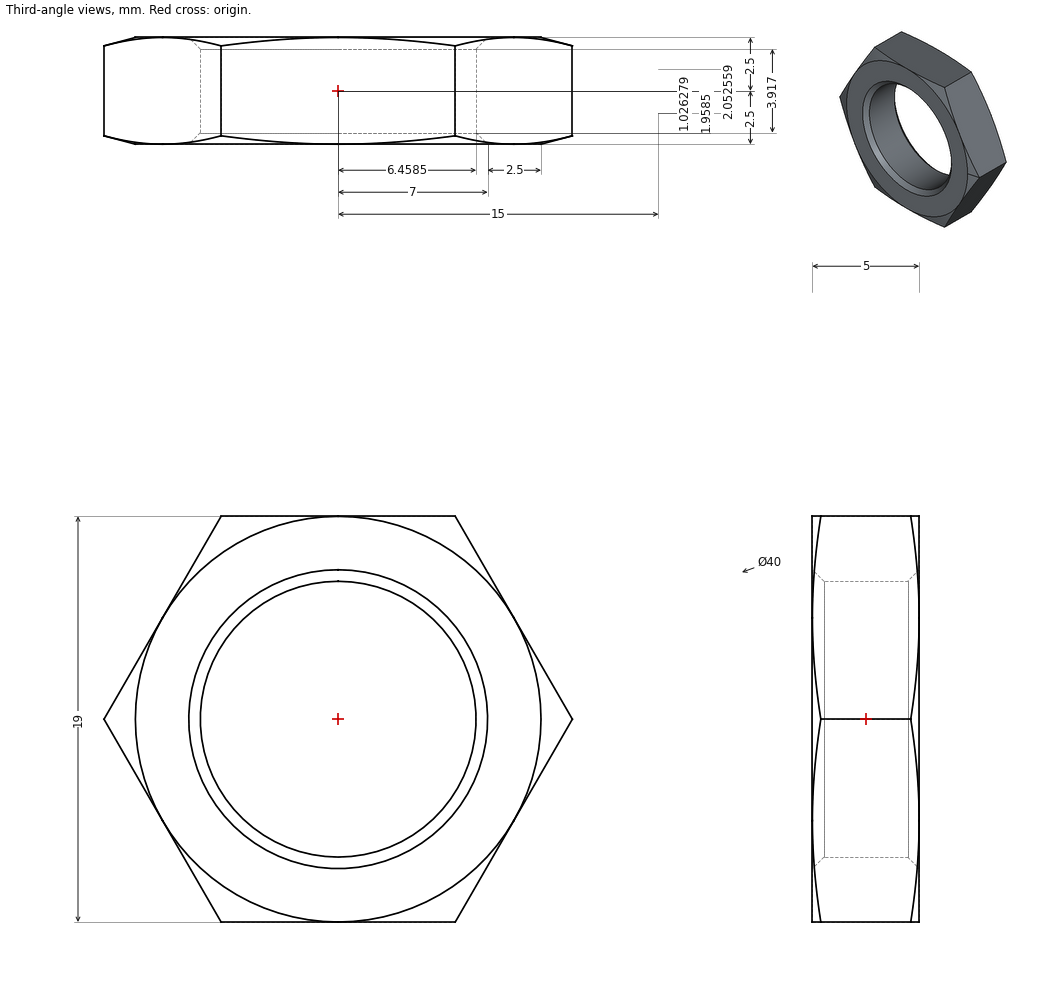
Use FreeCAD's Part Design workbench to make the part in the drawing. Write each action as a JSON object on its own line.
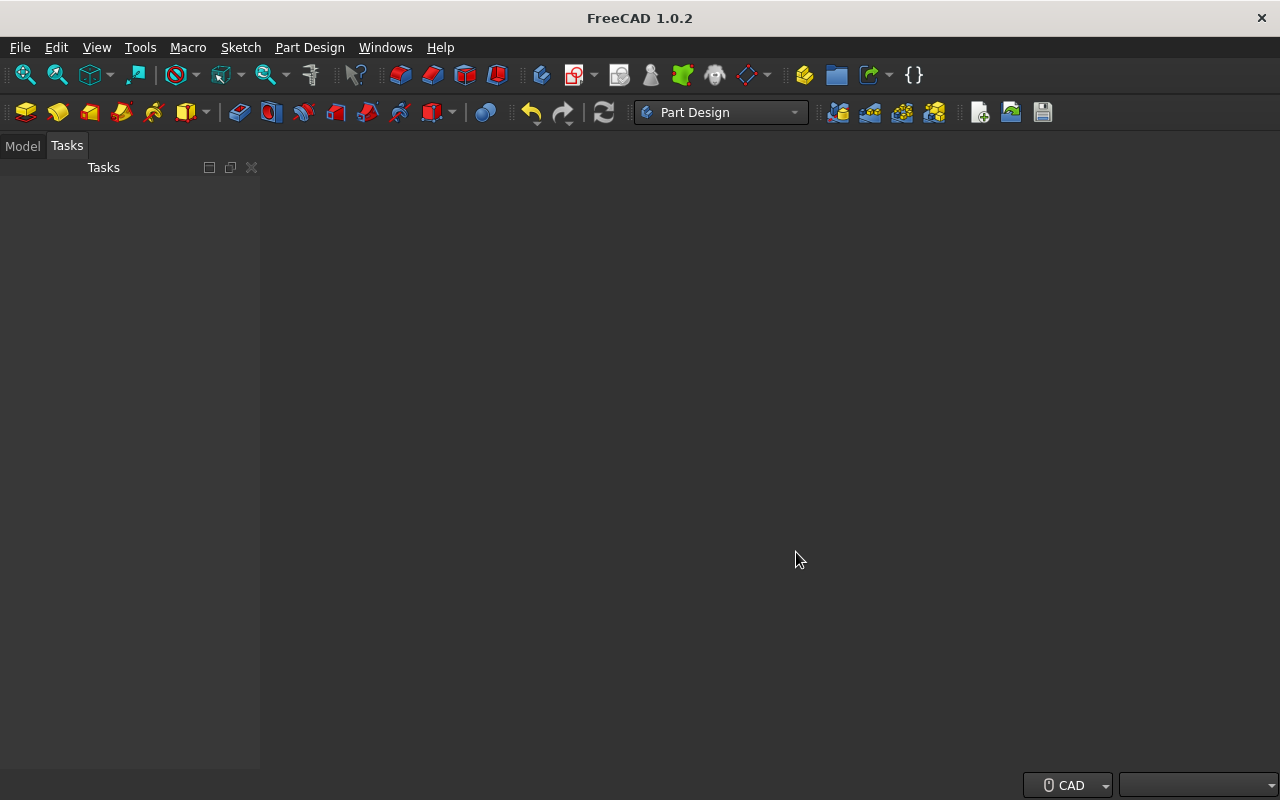
{"action": "key", "text": "ctrl+n"}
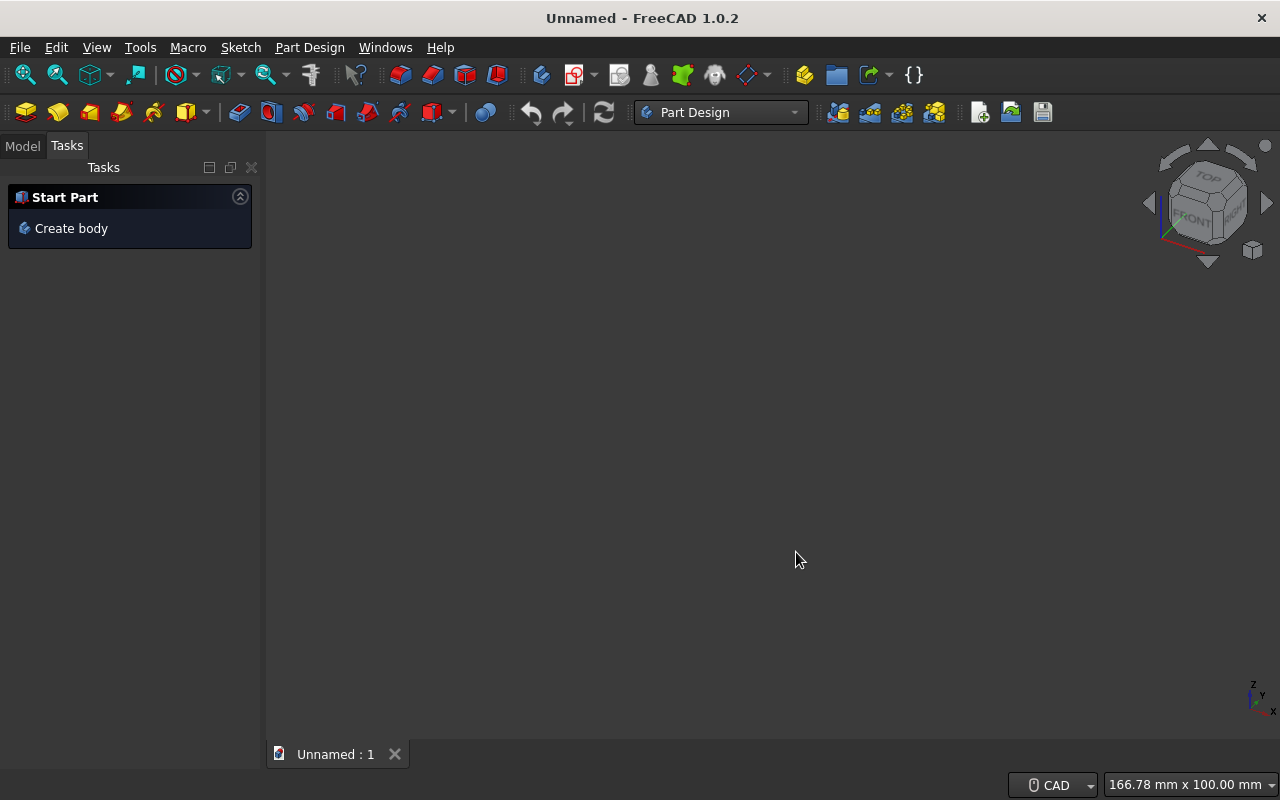
{"action": "left_click", "coordinate": [574, 76]}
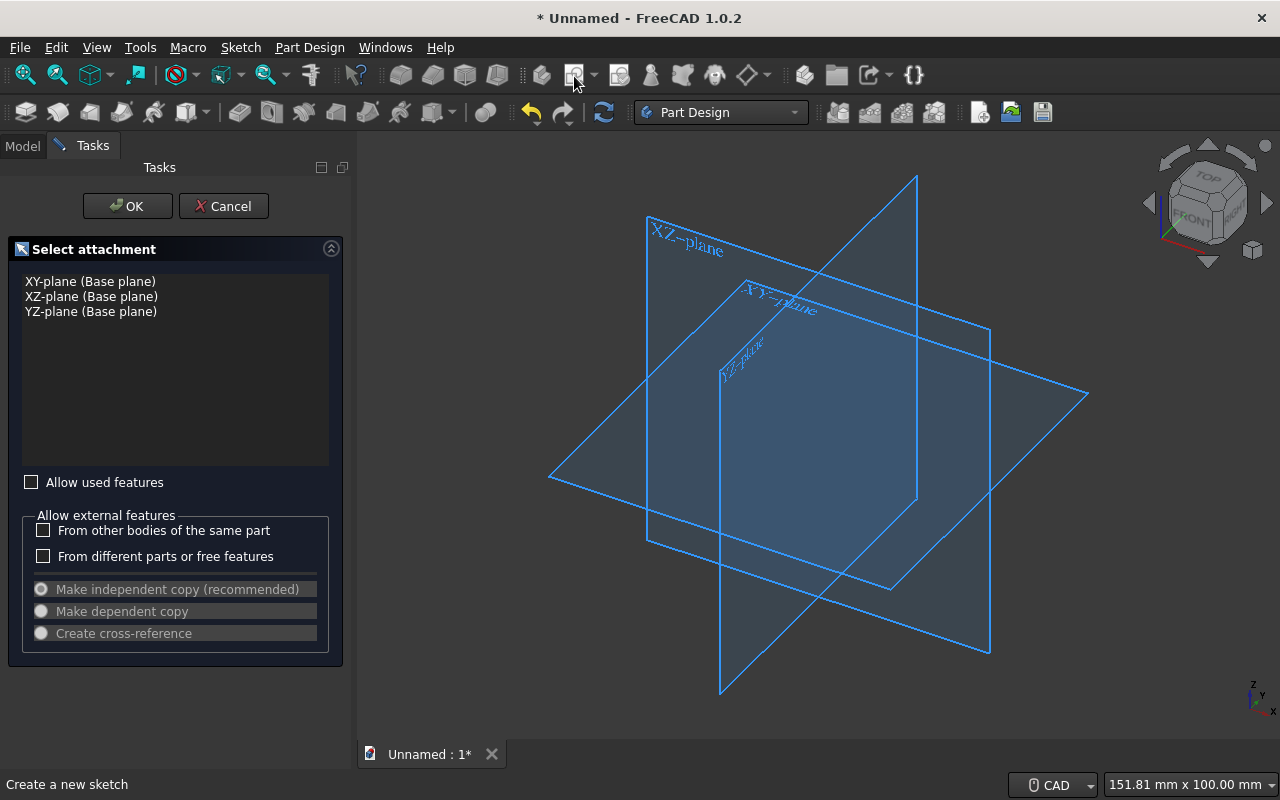
{"action": "left_click", "coordinate": [82, 282]}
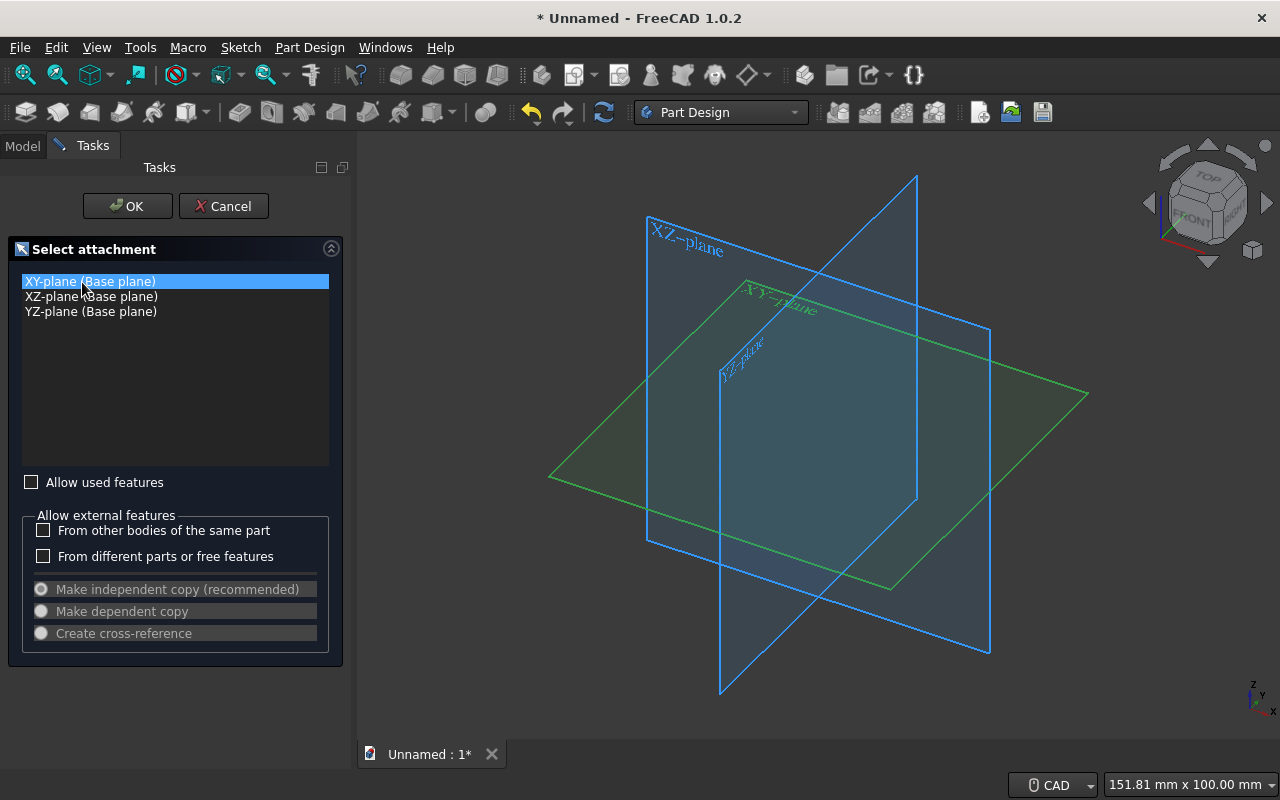
{"action": "left_click", "coordinate": [128, 206]}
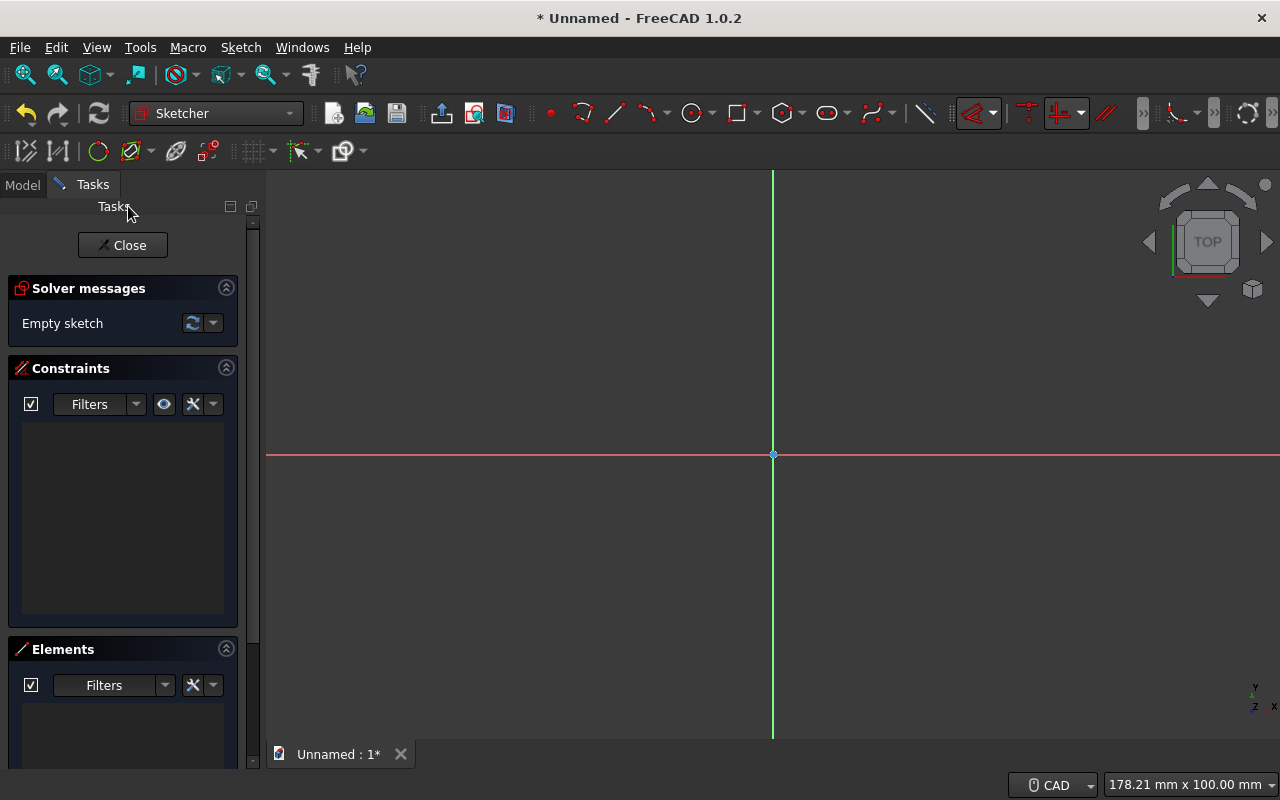
{"action": "scroll", "coordinate": [833, 454], "scroll_direction": "up", "scroll_amount": 10}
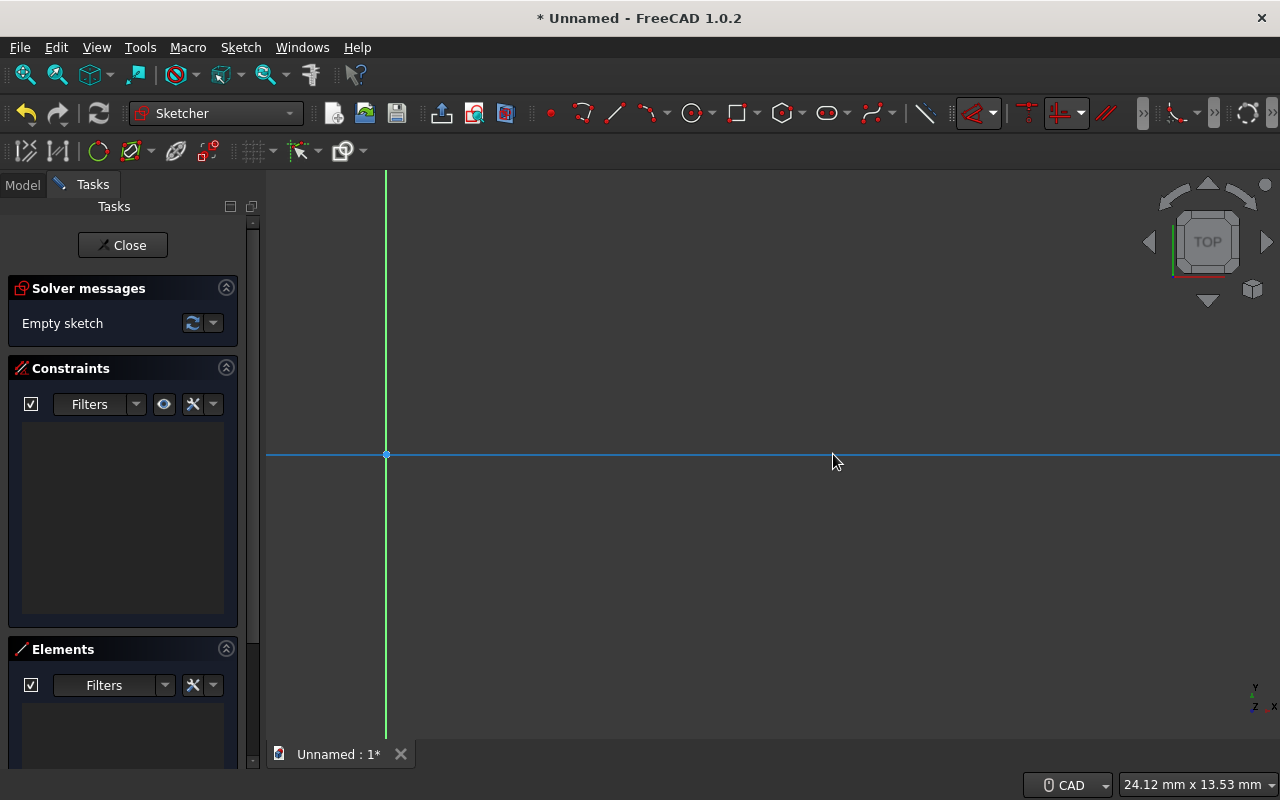
{"action": "left_click", "coordinate": [584, 114]}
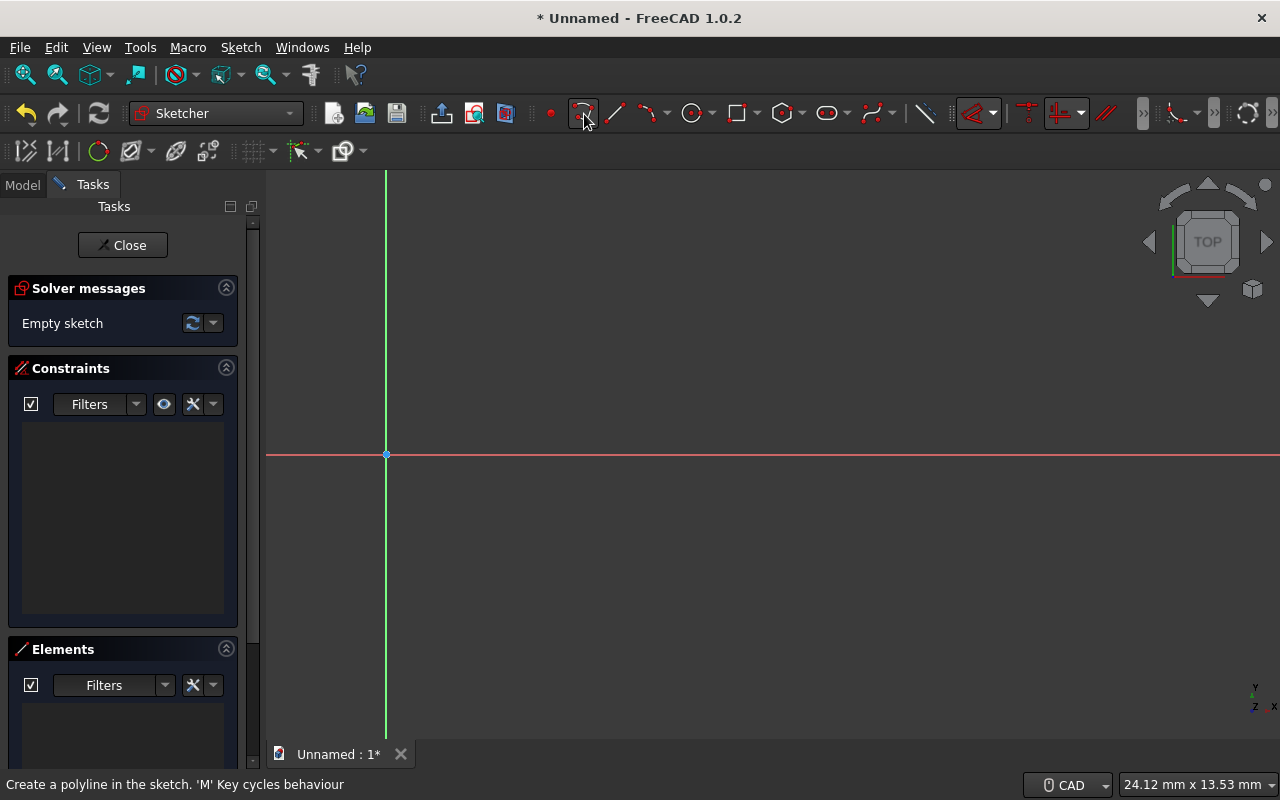
{"action": "left_click", "coordinate": [658, 537]}
{"action": "left_click", "coordinate": [680, 560]}
{"action": "left_click", "coordinate": [785, 560]}
{"action": "left_click", "coordinate": [1017, 498]}
{"action": "left_click", "coordinate": [1017, 411]}
{"action": "left_click", "coordinate": [785, 349]}
{"action": "left_click", "coordinate": [680, 349]}
{"action": "left_click", "coordinate": [658, 372]}
{"action": "left_click", "coordinate": [658, 538]}
{"action": "key", "text": "Escape"}
{"action": "key", "text": "Escape"}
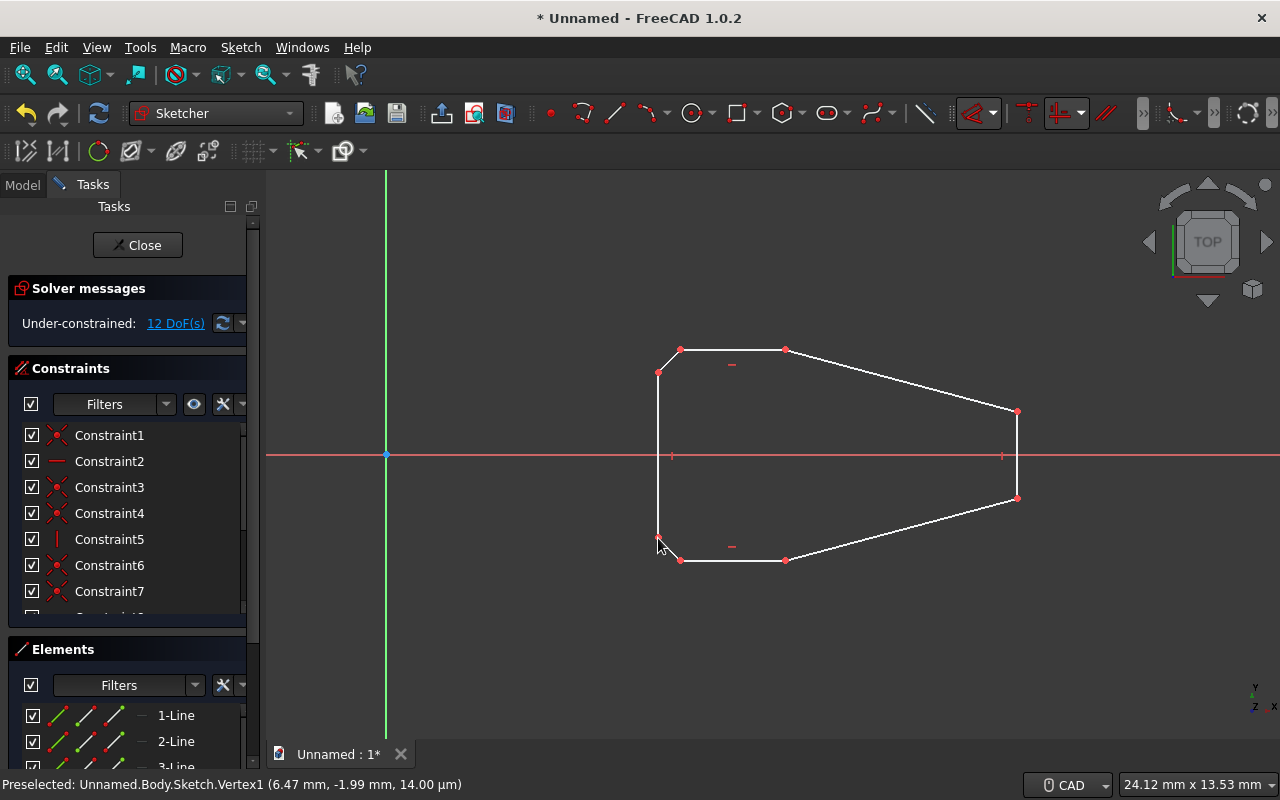
{"action": "left_click", "coordinate": [972, 114]}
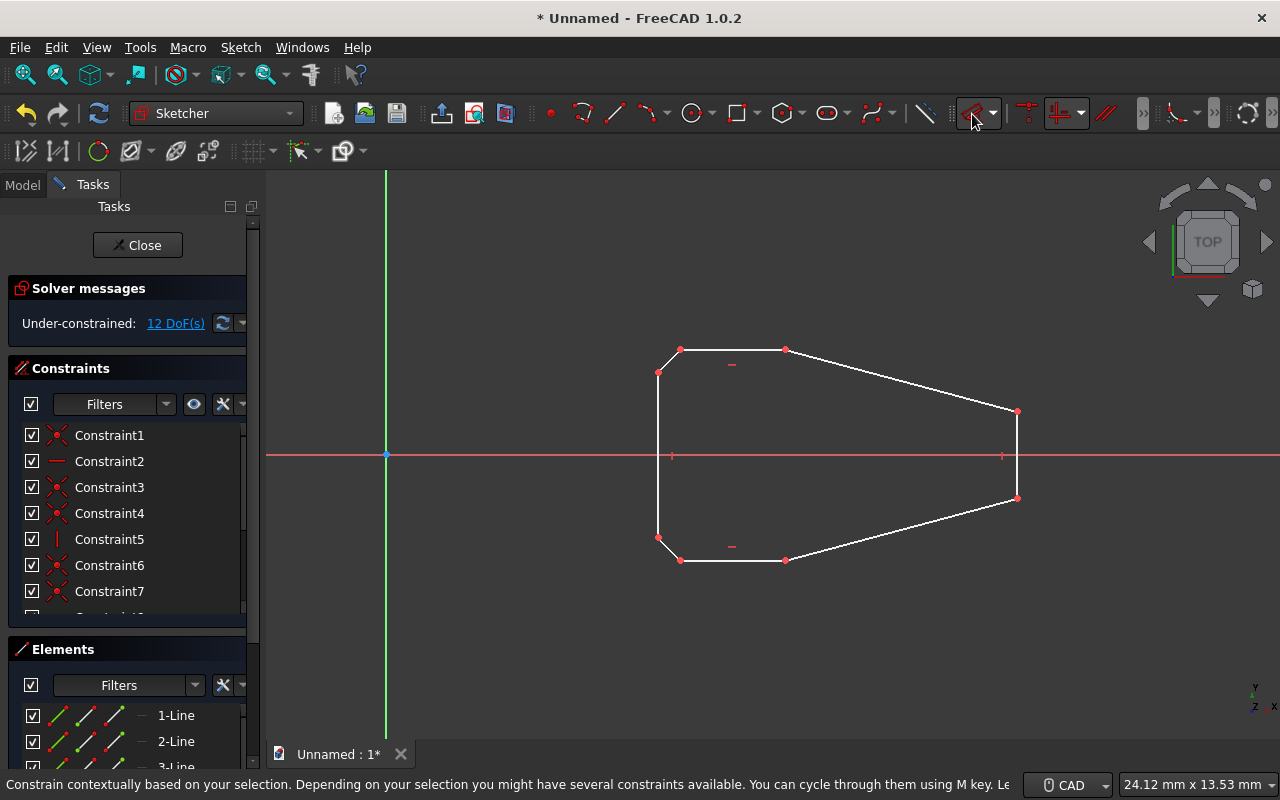
{"action": "left_click", "coordinate": [680, 561]}
{"action": "left_click", "coordinate": [533, 595]}